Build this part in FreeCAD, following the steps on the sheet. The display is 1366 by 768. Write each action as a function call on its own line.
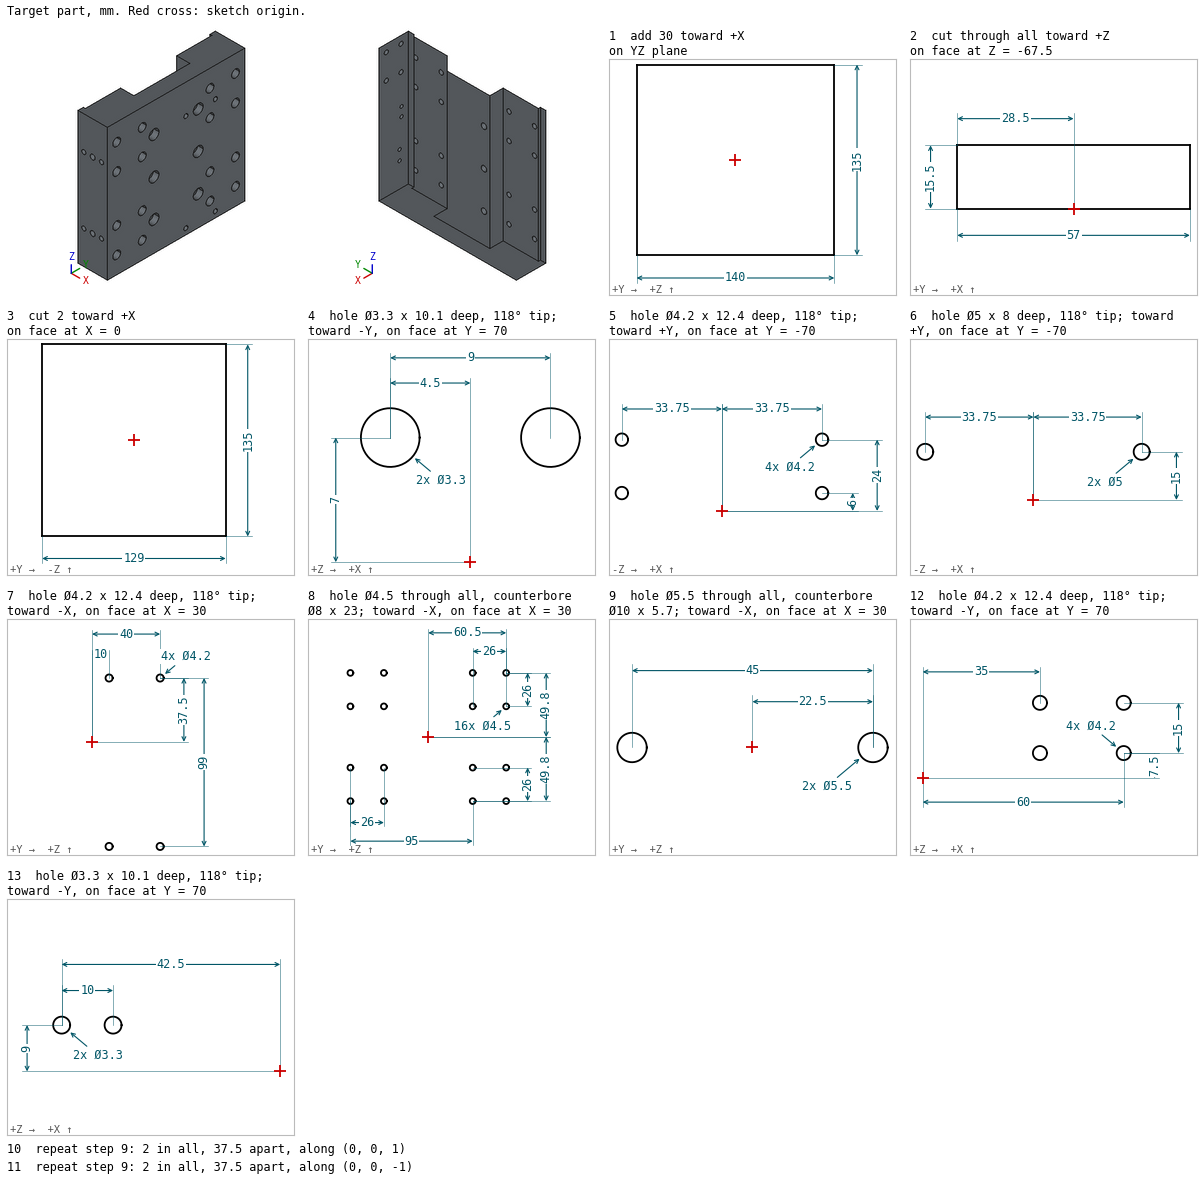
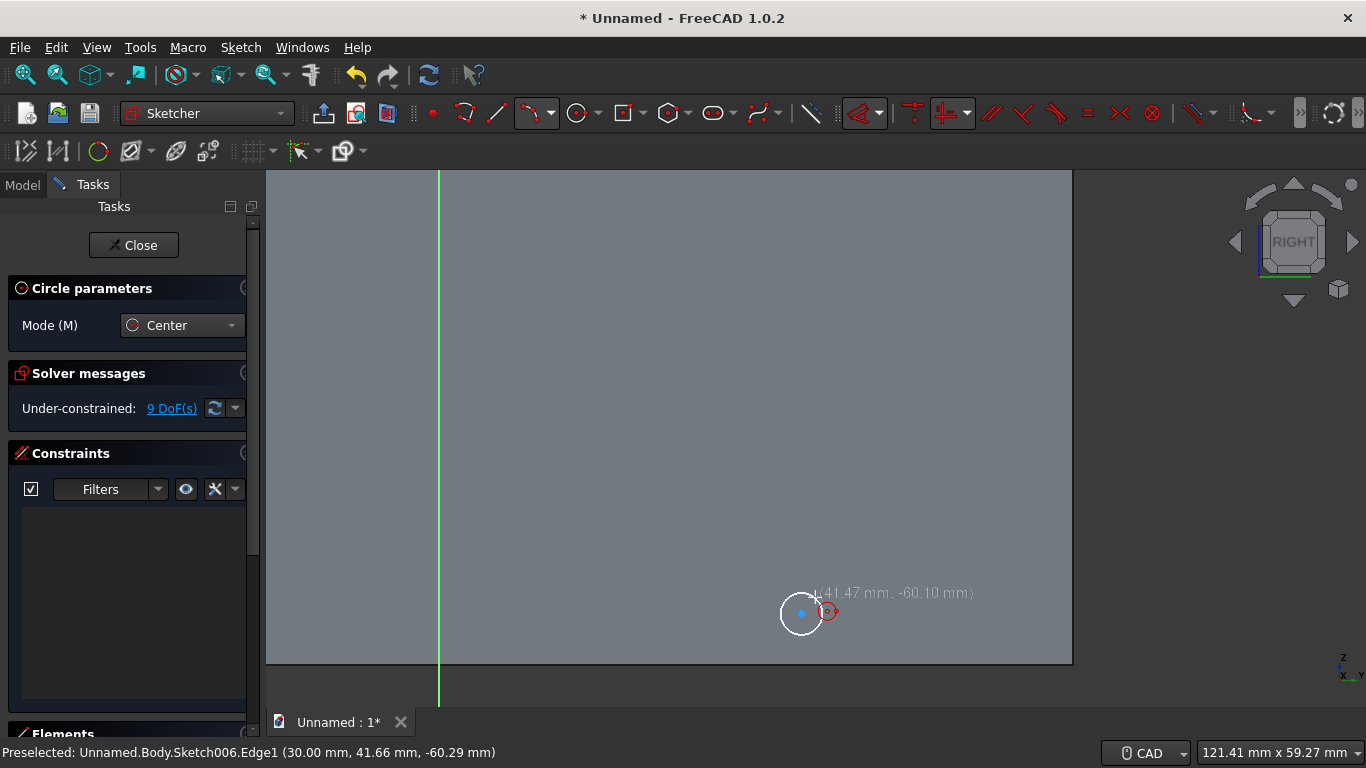
click(530, 611)
click(543, 597)
key(Escape)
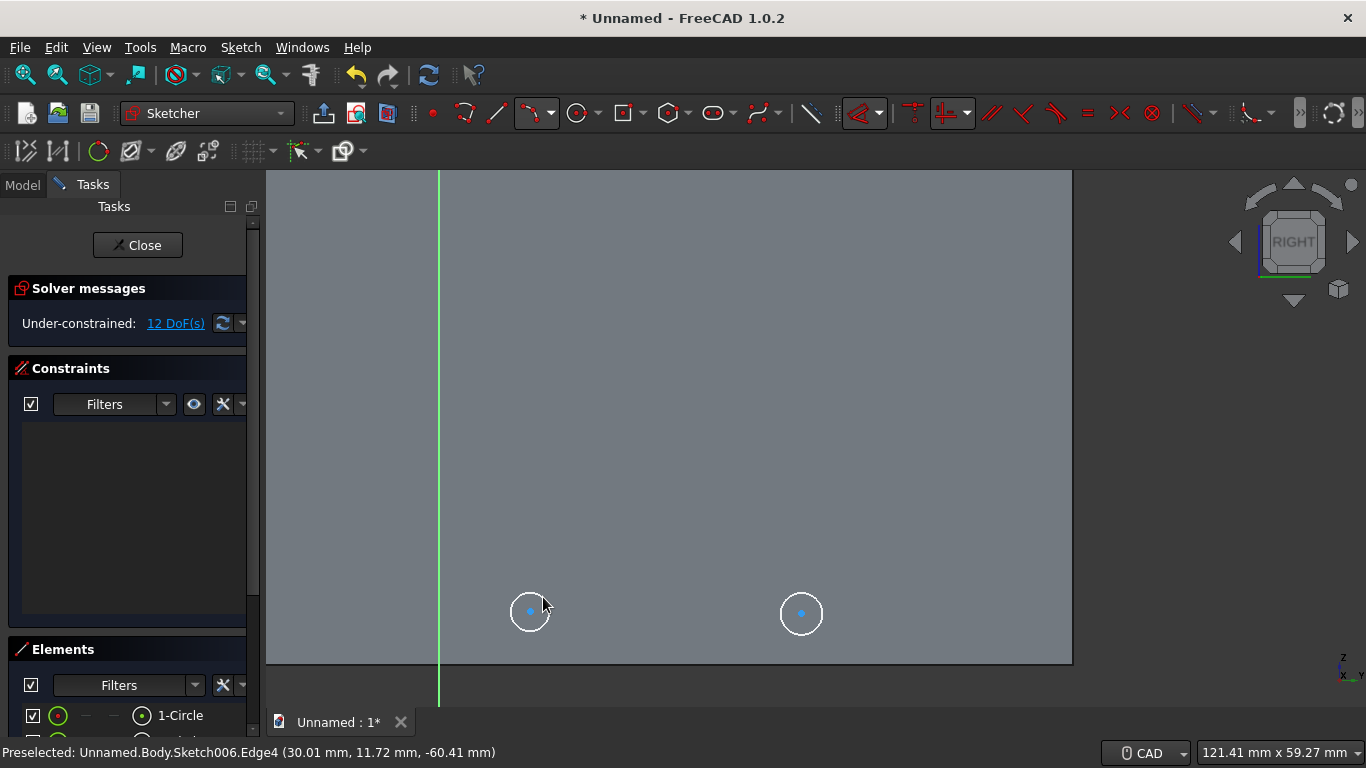
scroll(816, 599, down, 5)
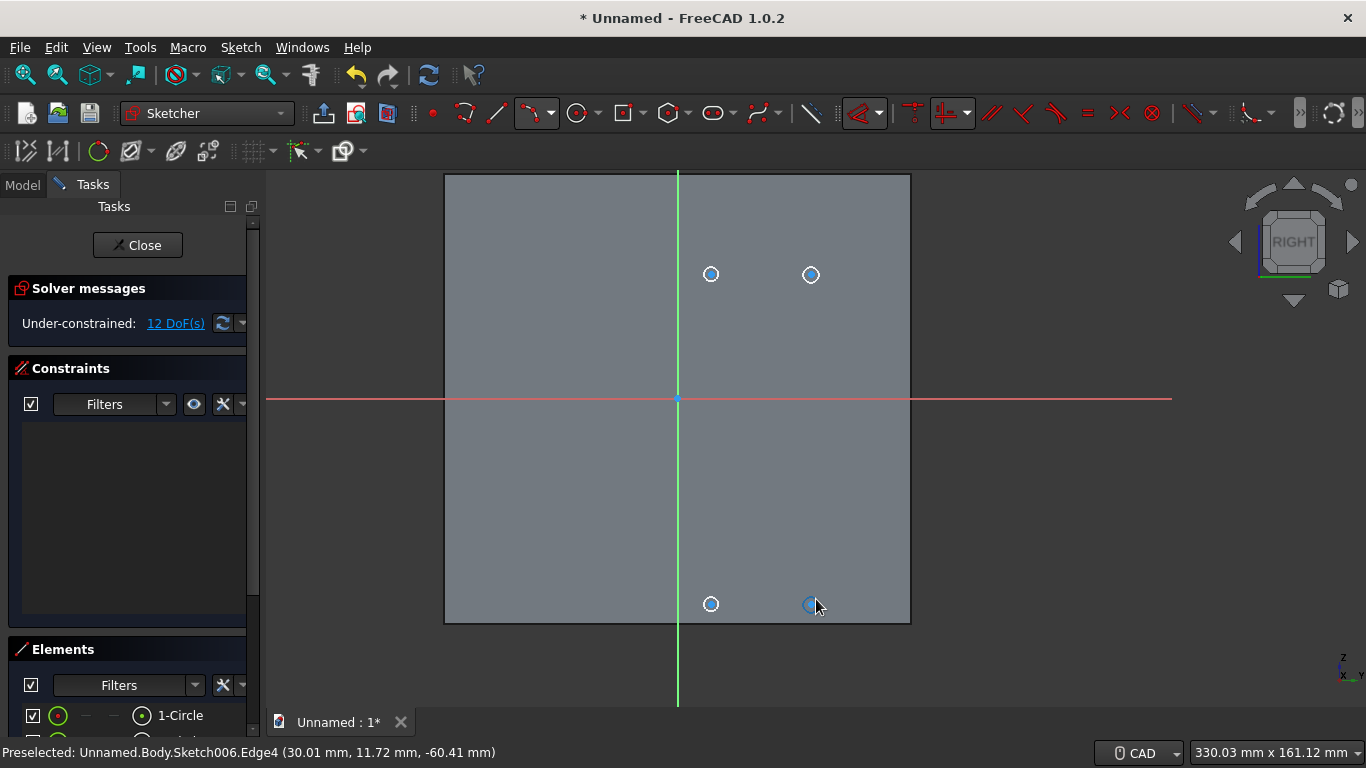
scroll(816, 270, up, 3)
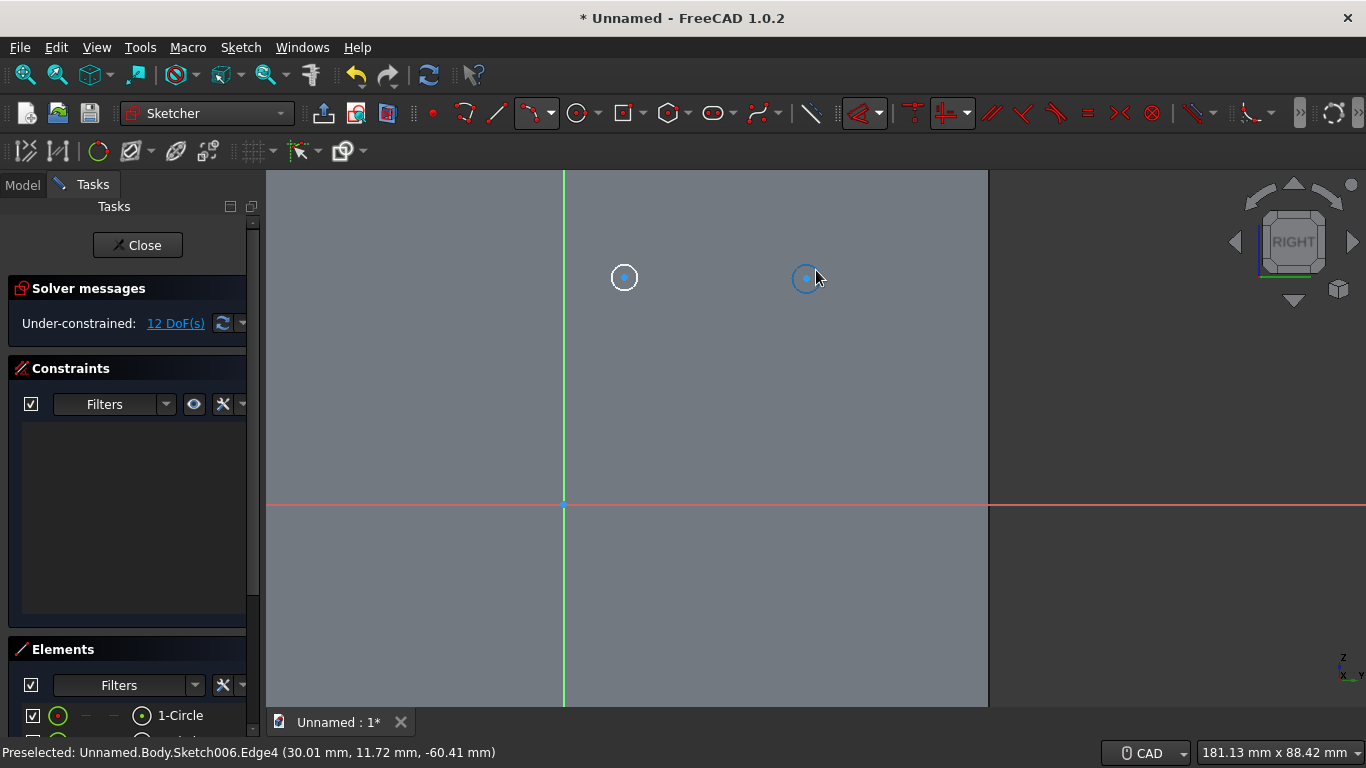
click(816, 269)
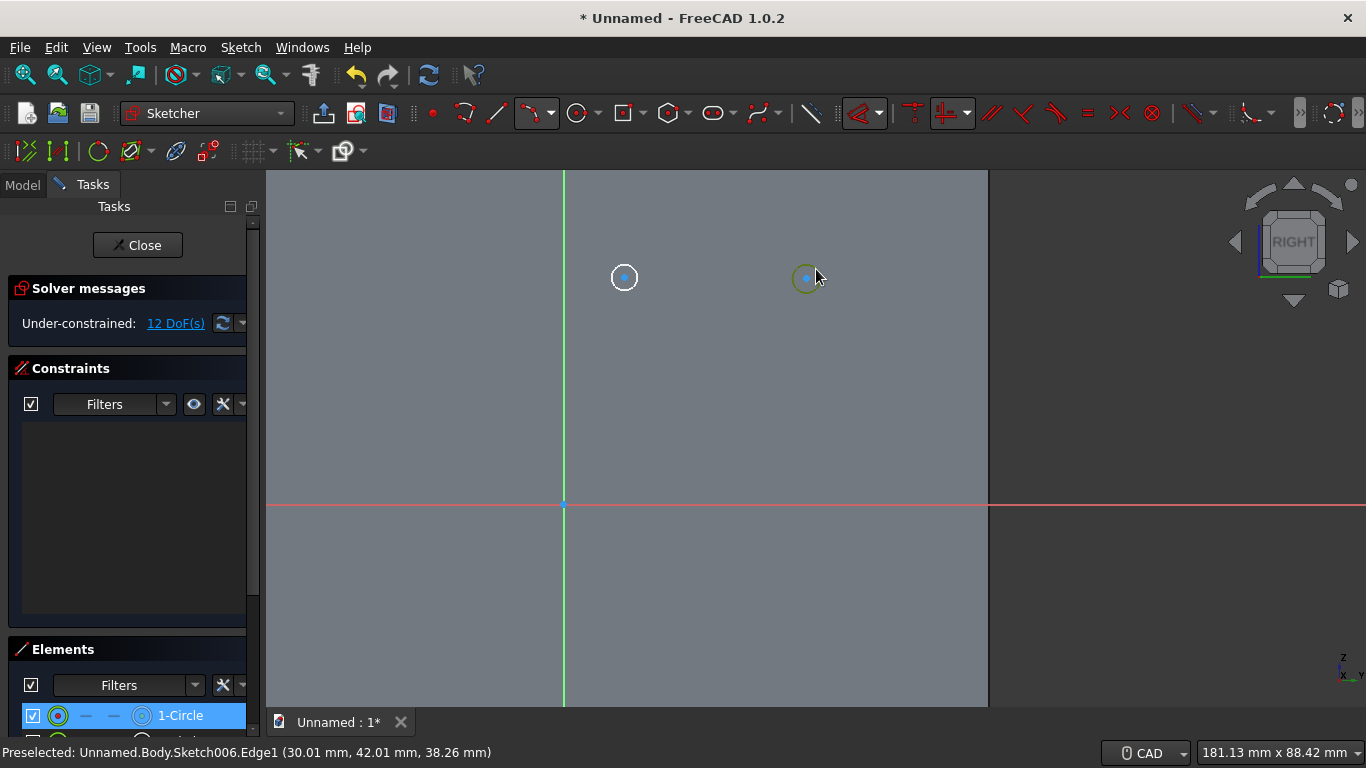
click(633, 269)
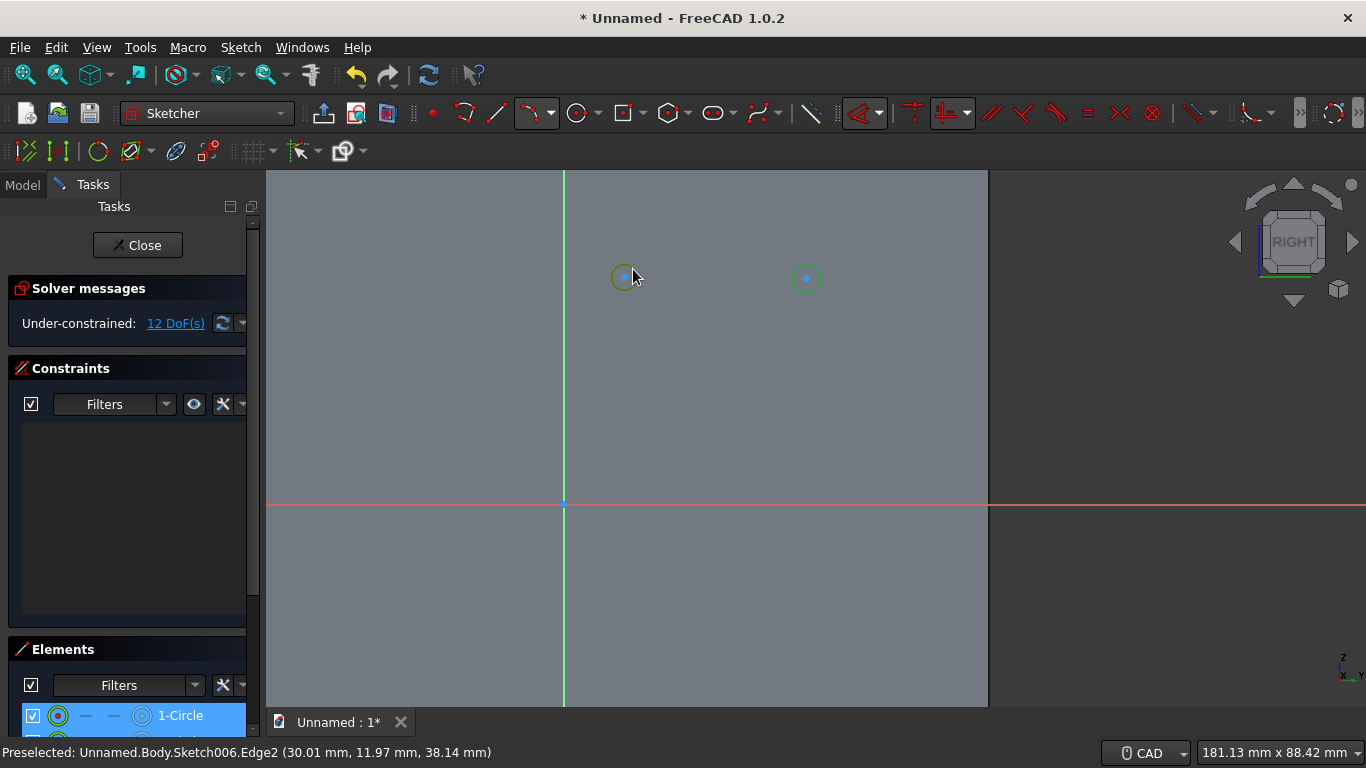
scroll(816, 269, down, 3)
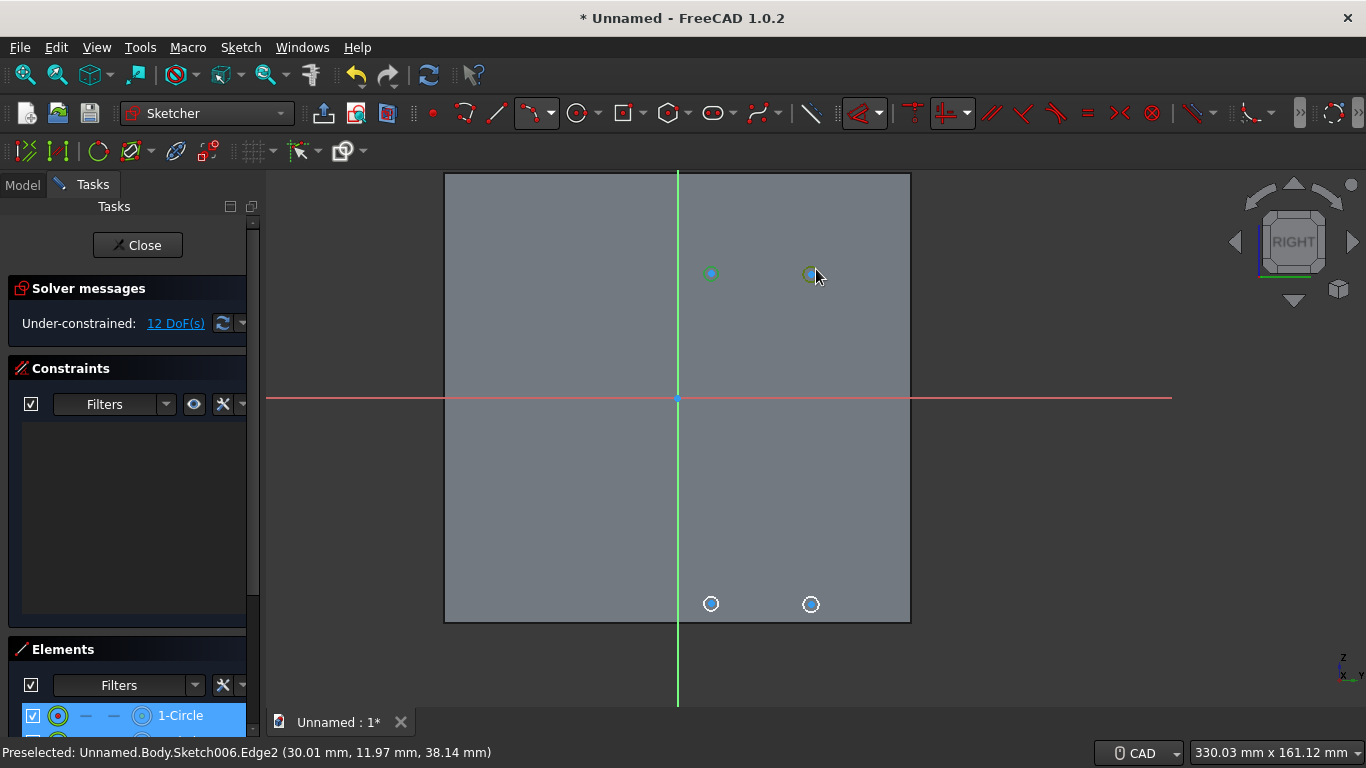
scroll(816, 599, up, 3)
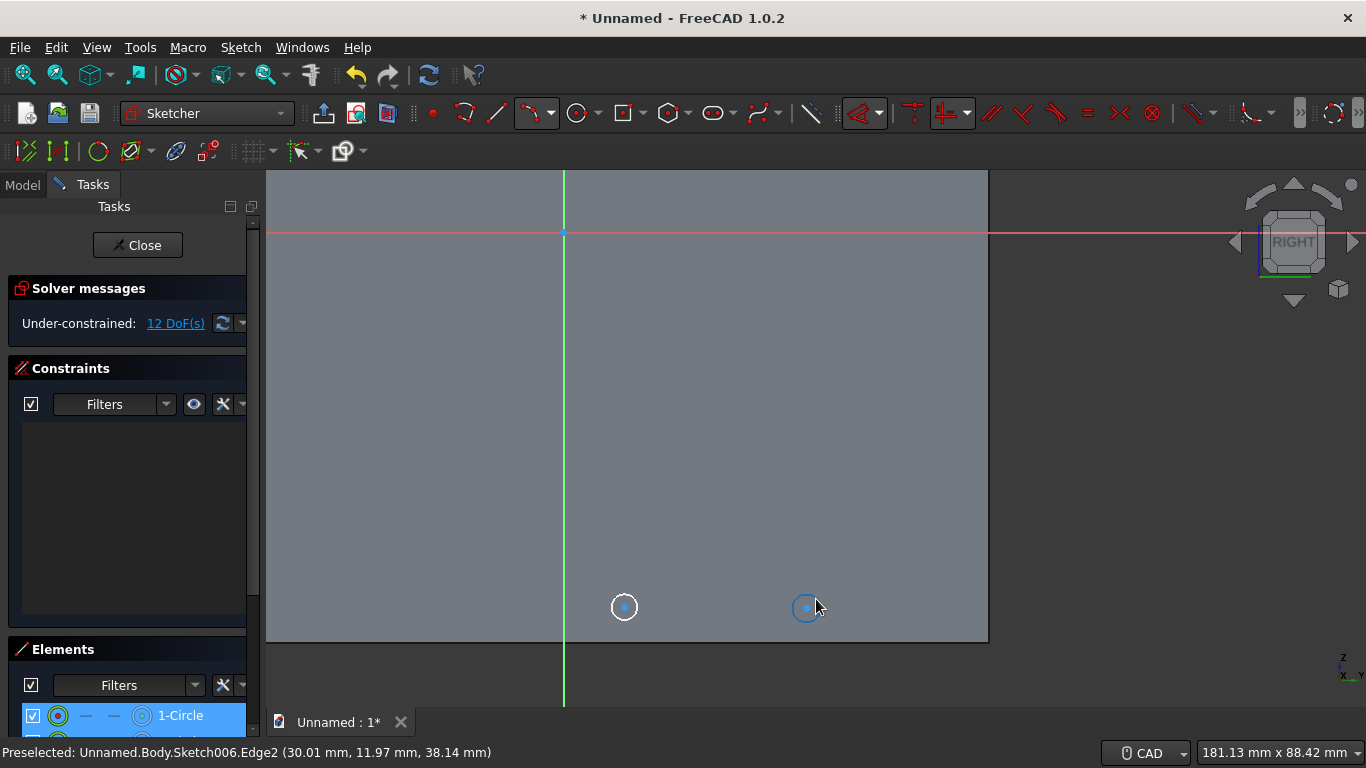
click(816, 599)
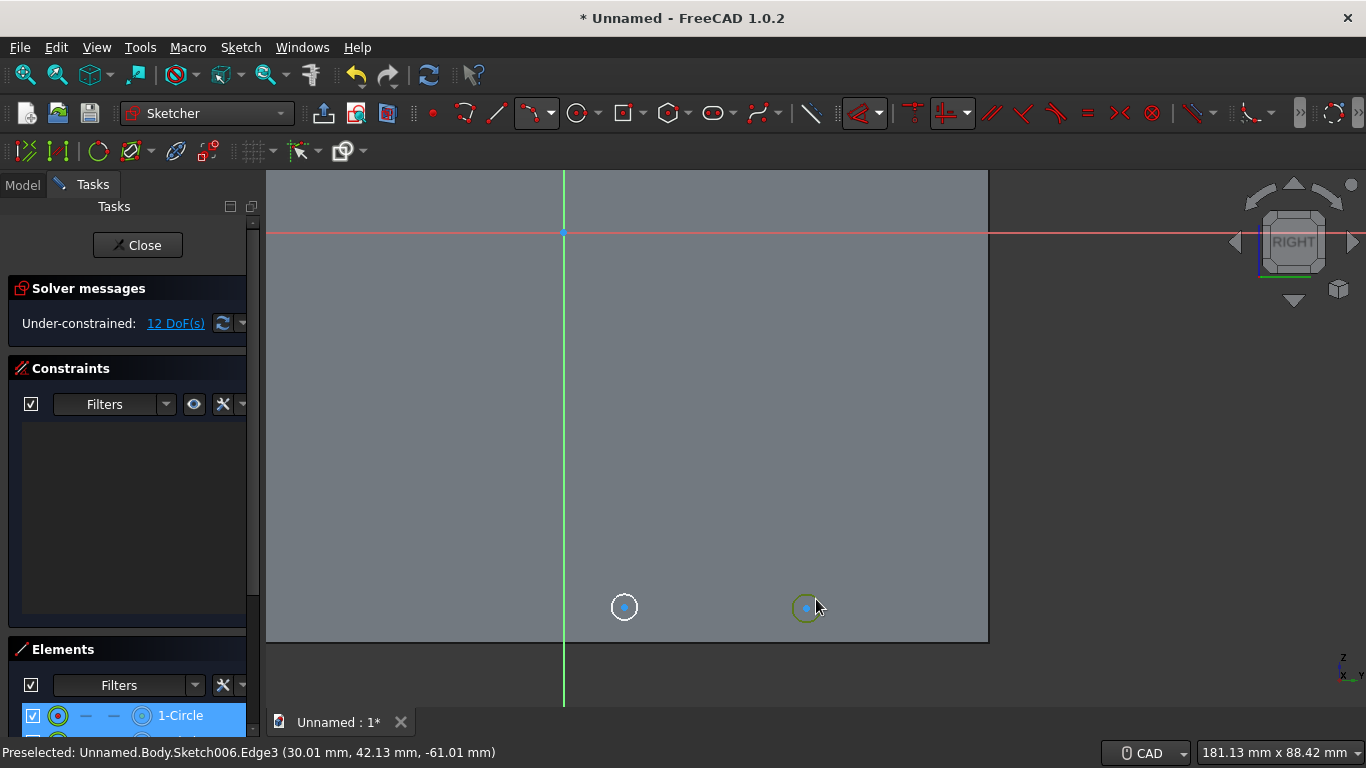
click(633, 598)